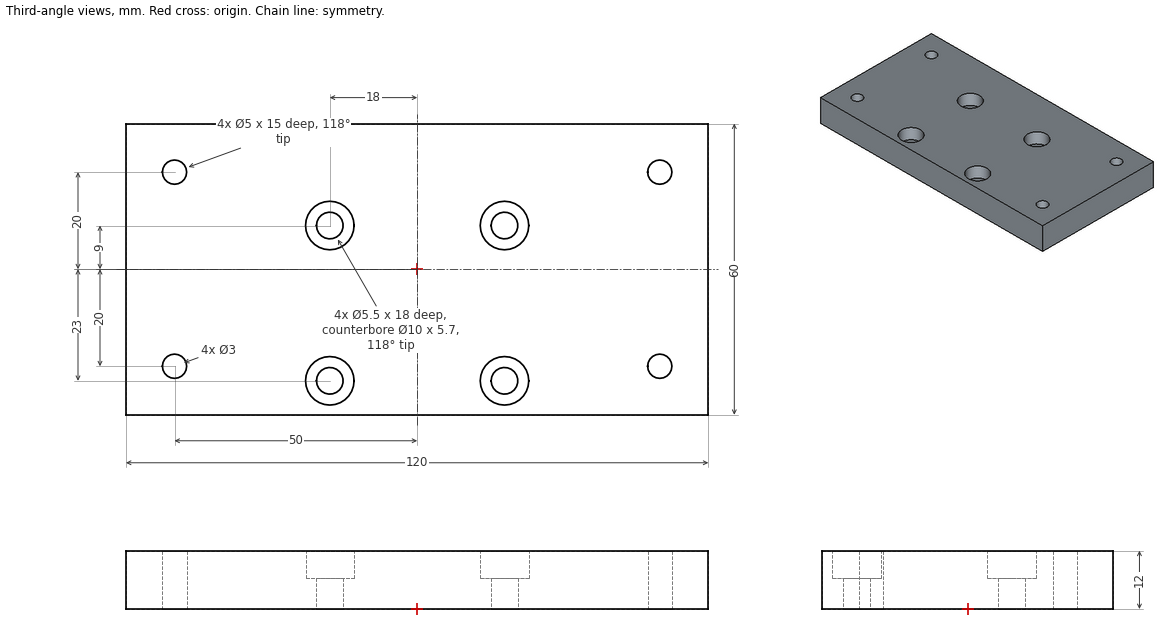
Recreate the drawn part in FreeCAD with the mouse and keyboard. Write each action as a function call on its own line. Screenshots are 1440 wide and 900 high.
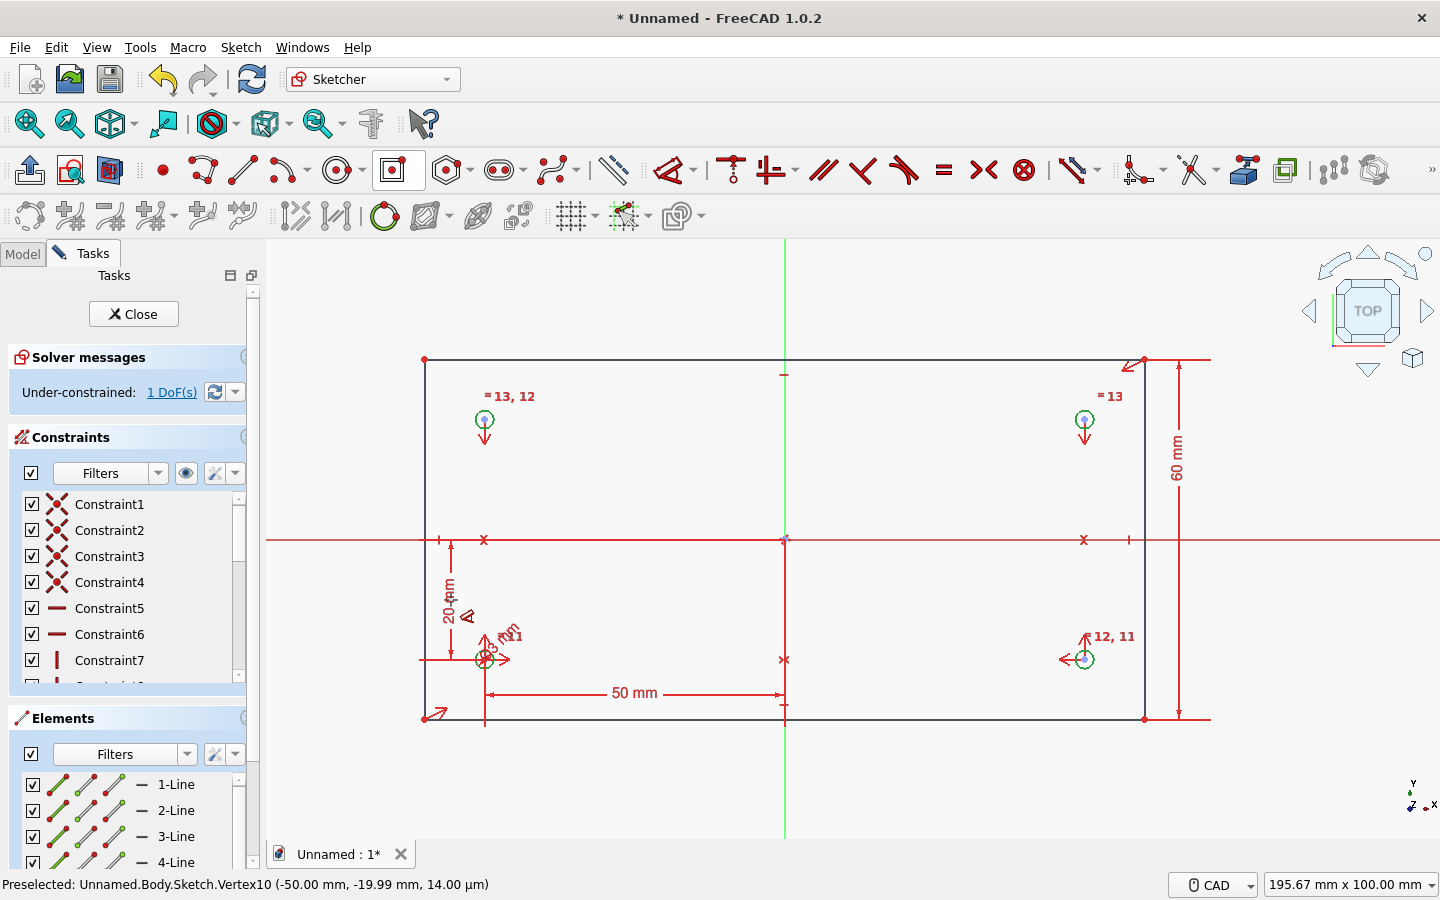
click(641, 720)
click(619, 754)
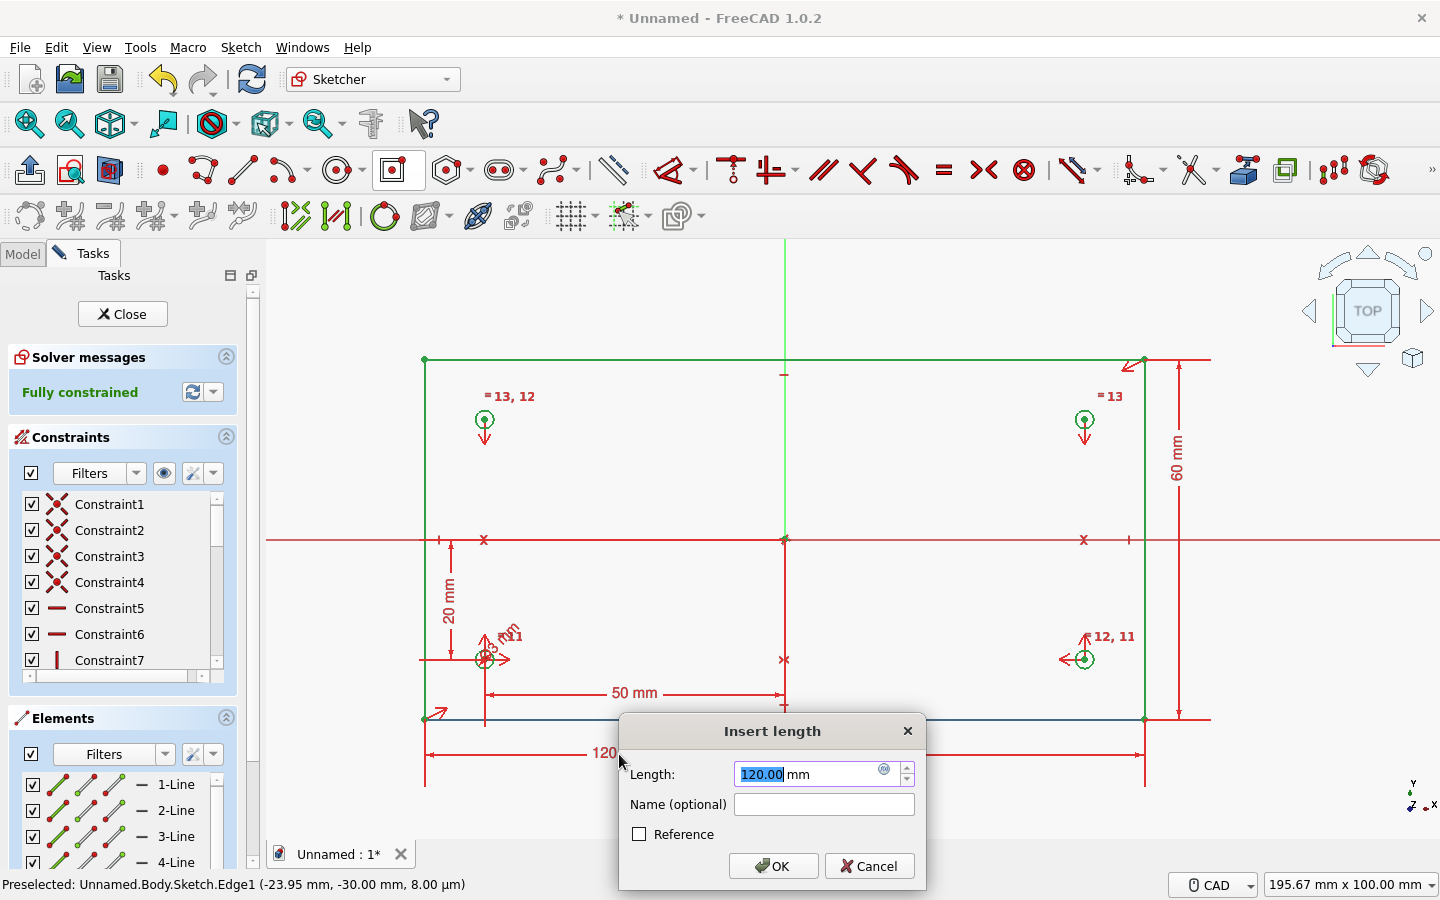
text(120)
key(Return)
key(Escape)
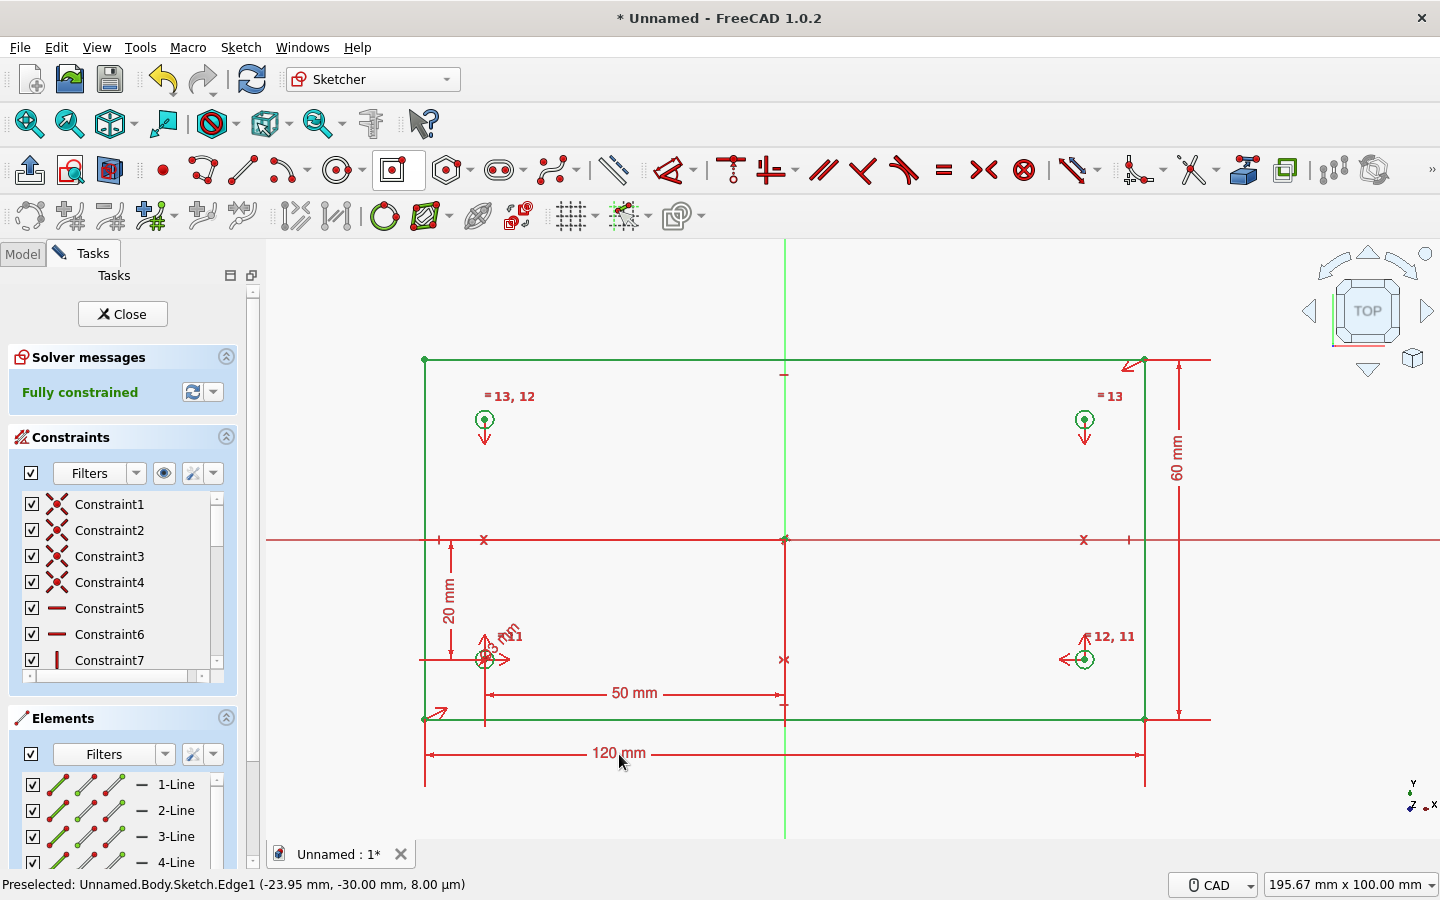
click(123, 314)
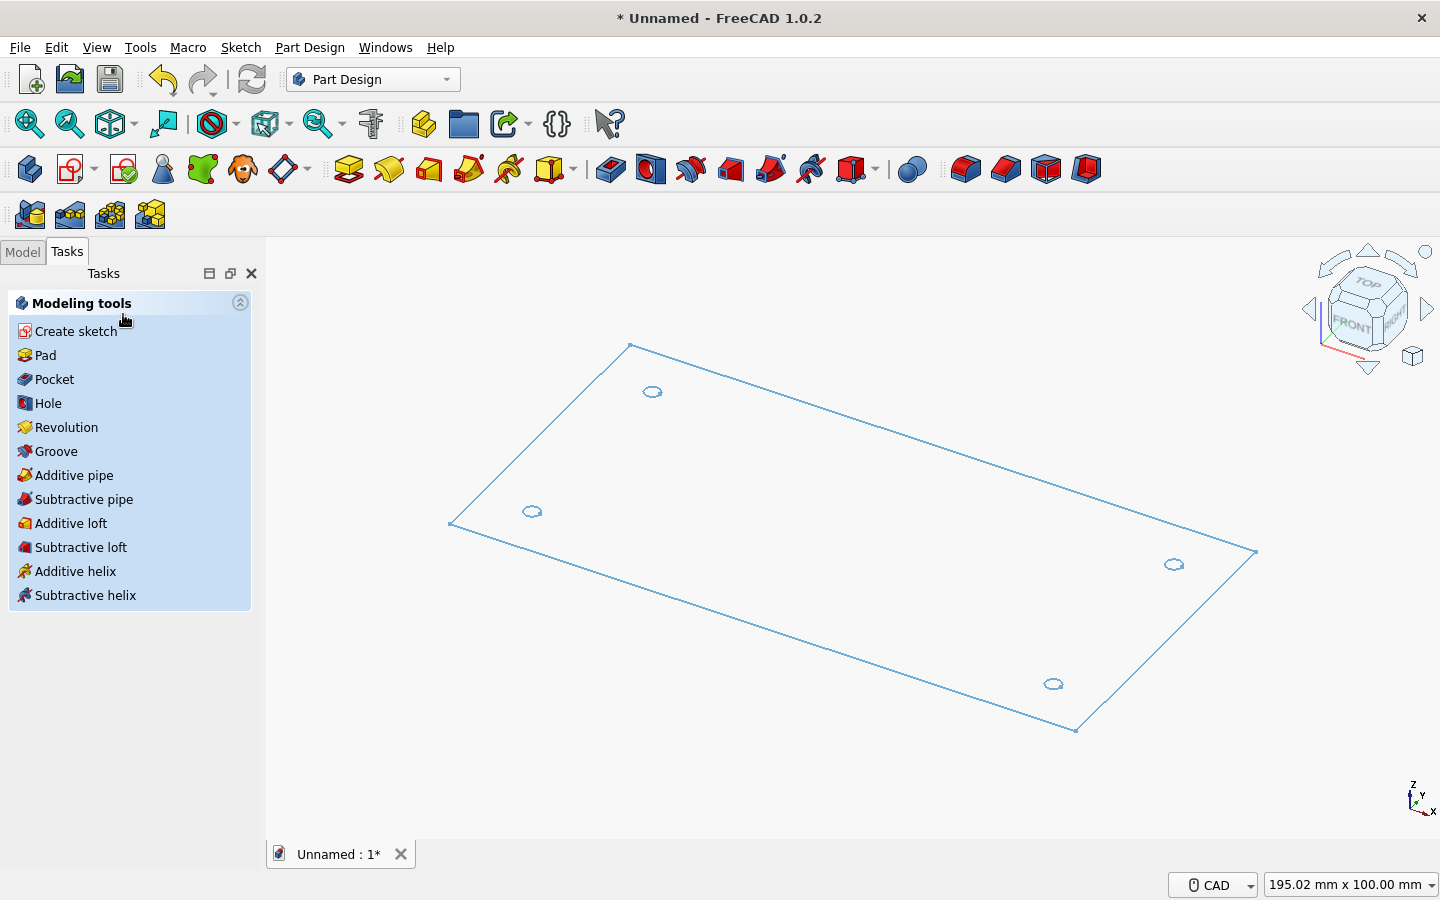
click(350, 170)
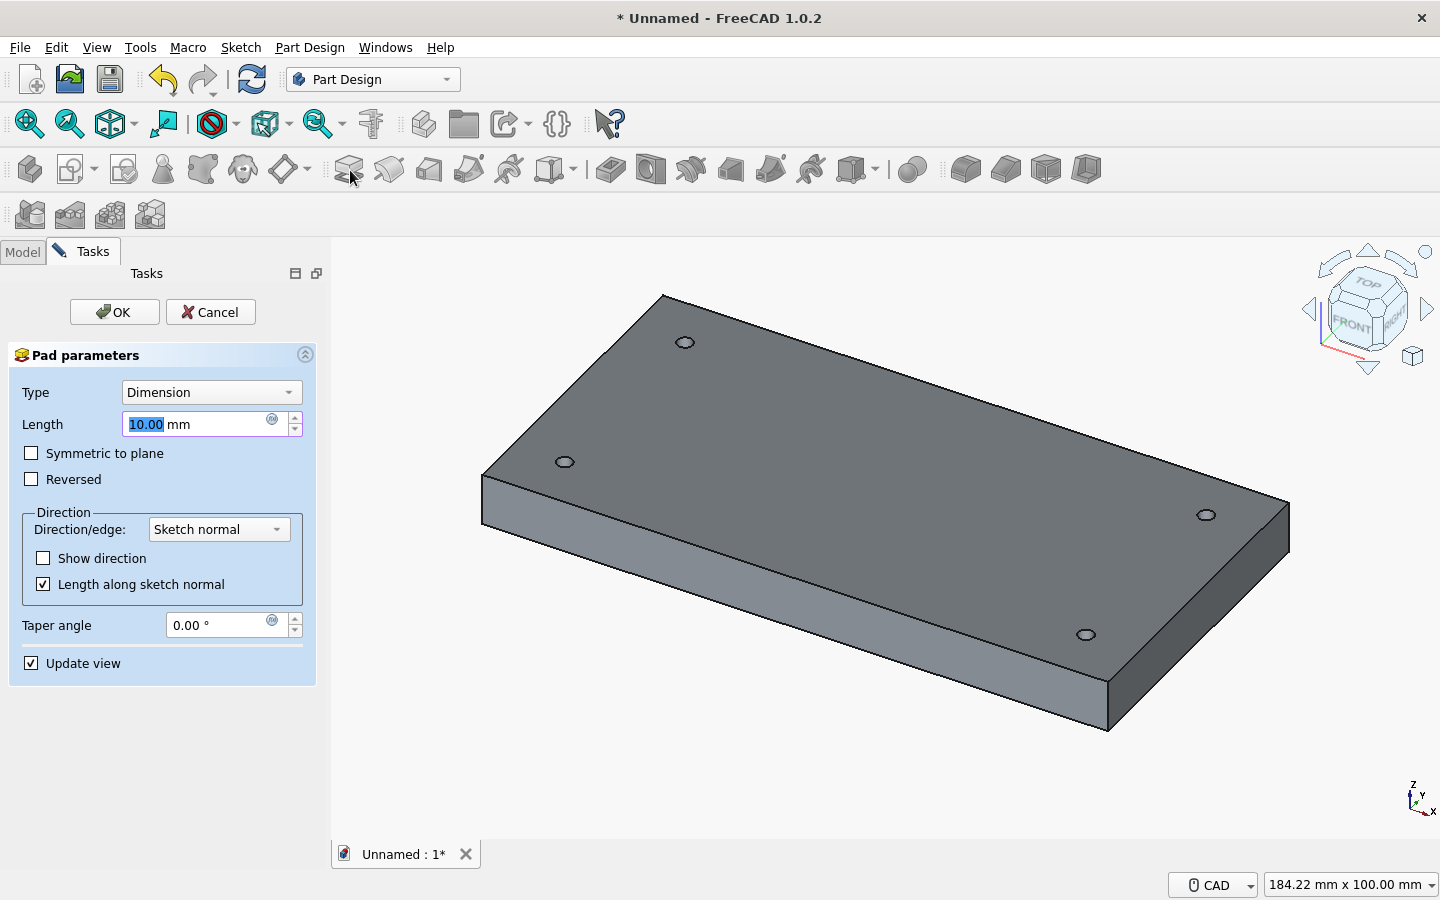
text(12)
key(Tab)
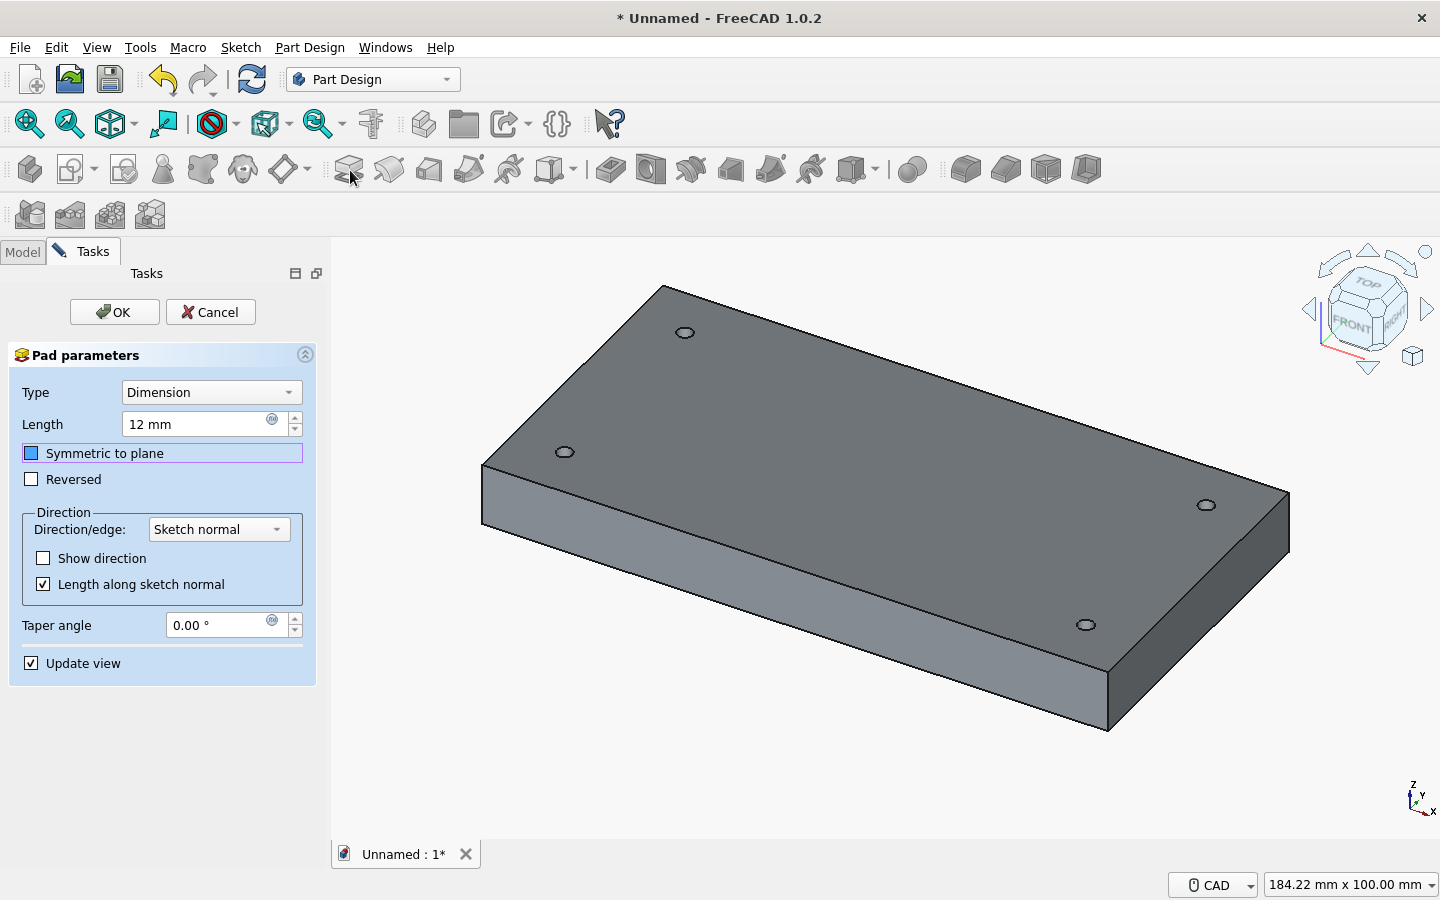
click(115, 312)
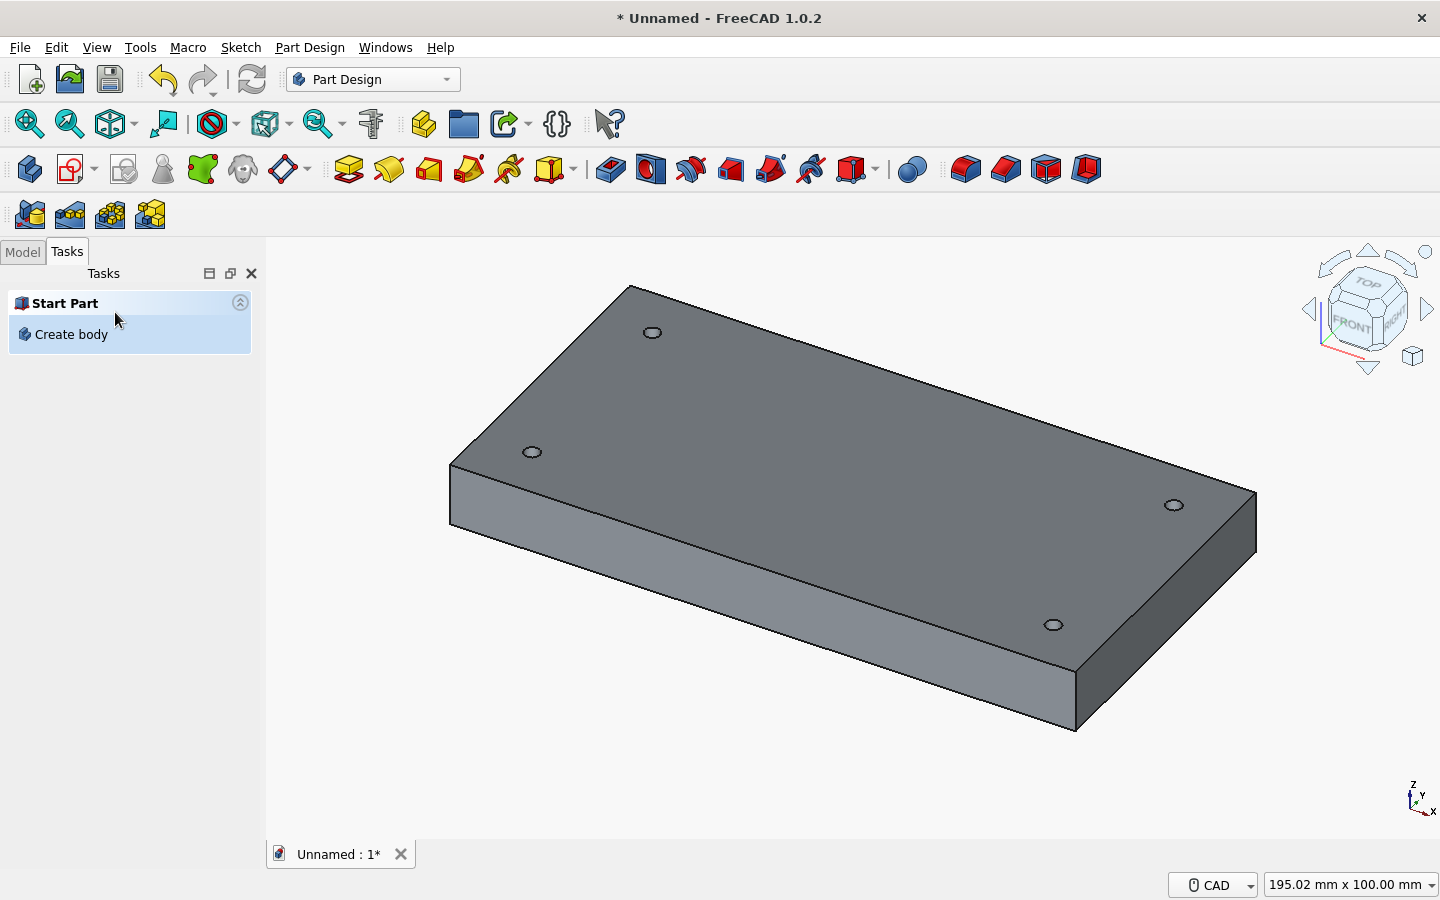
click(942, 507)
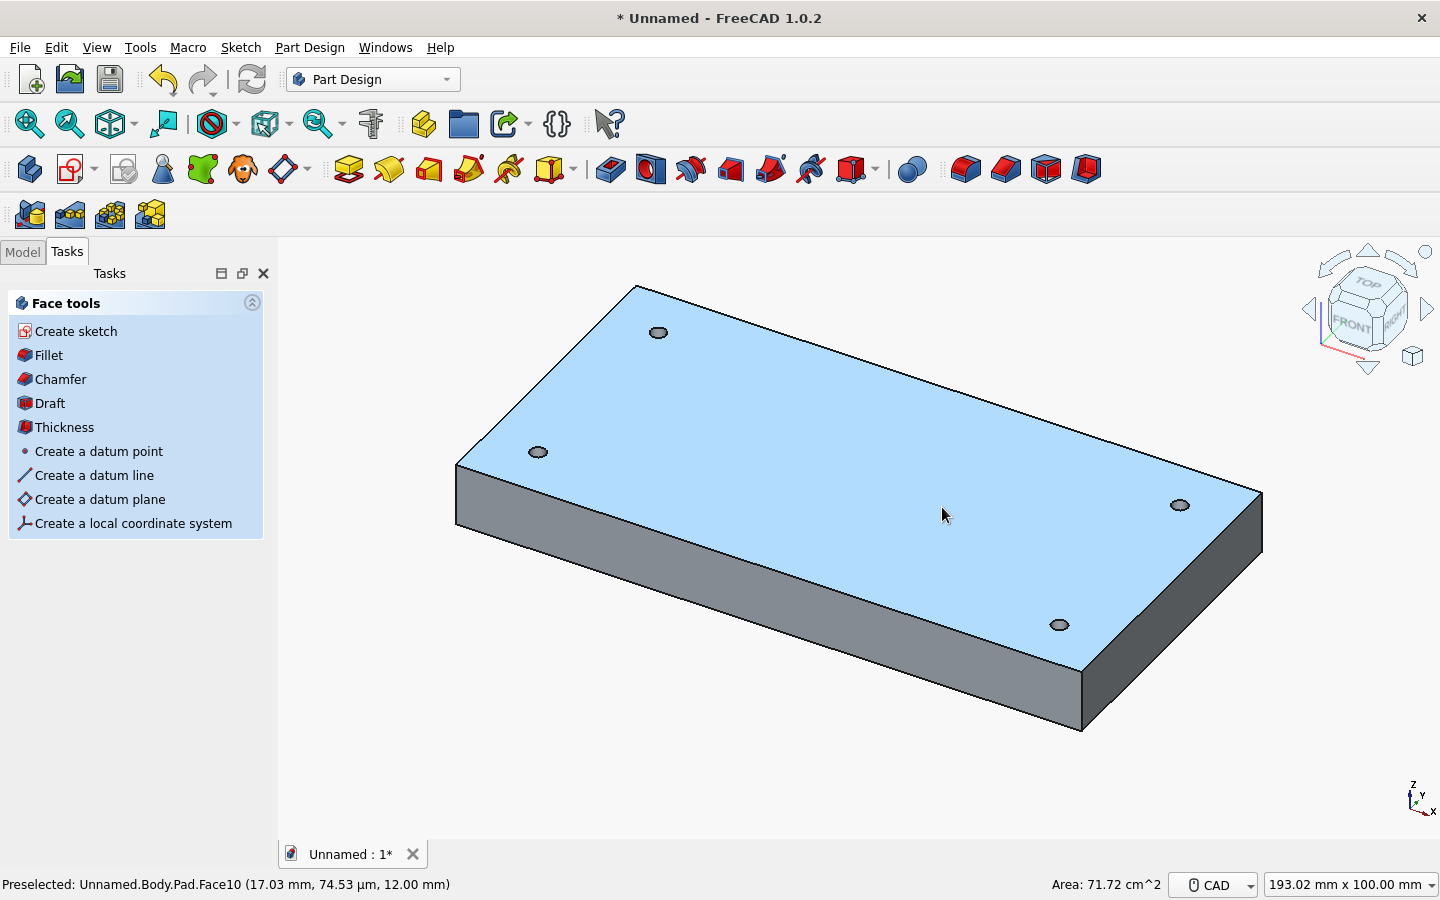
click(70, 170)